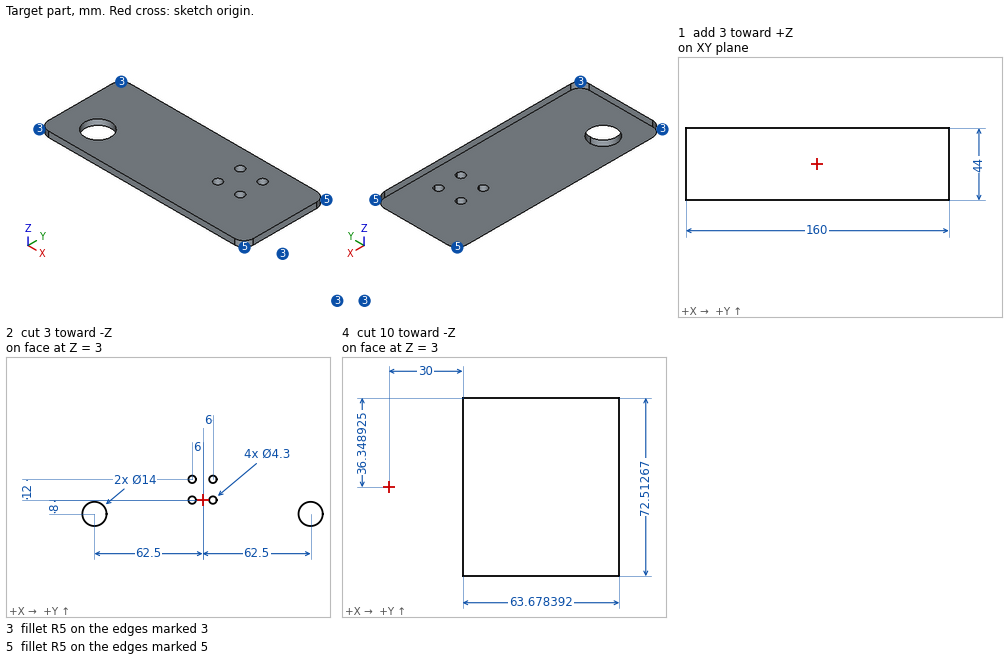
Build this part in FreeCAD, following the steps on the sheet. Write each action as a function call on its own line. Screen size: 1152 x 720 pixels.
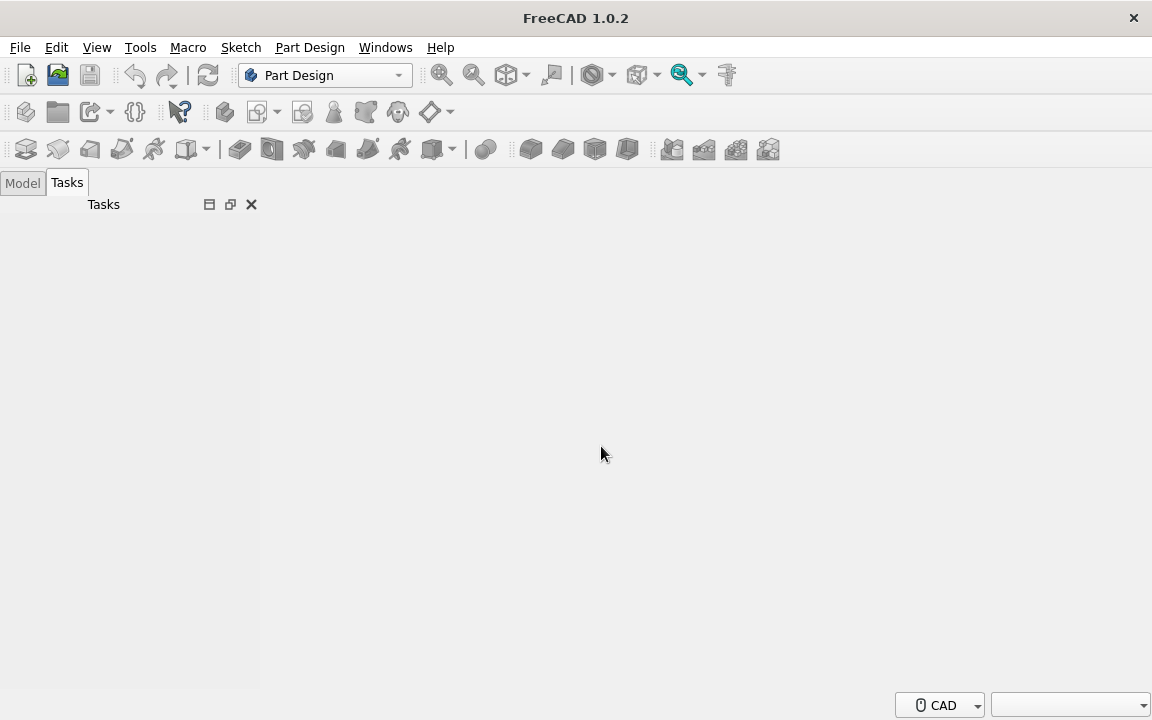
key(ctrl+n)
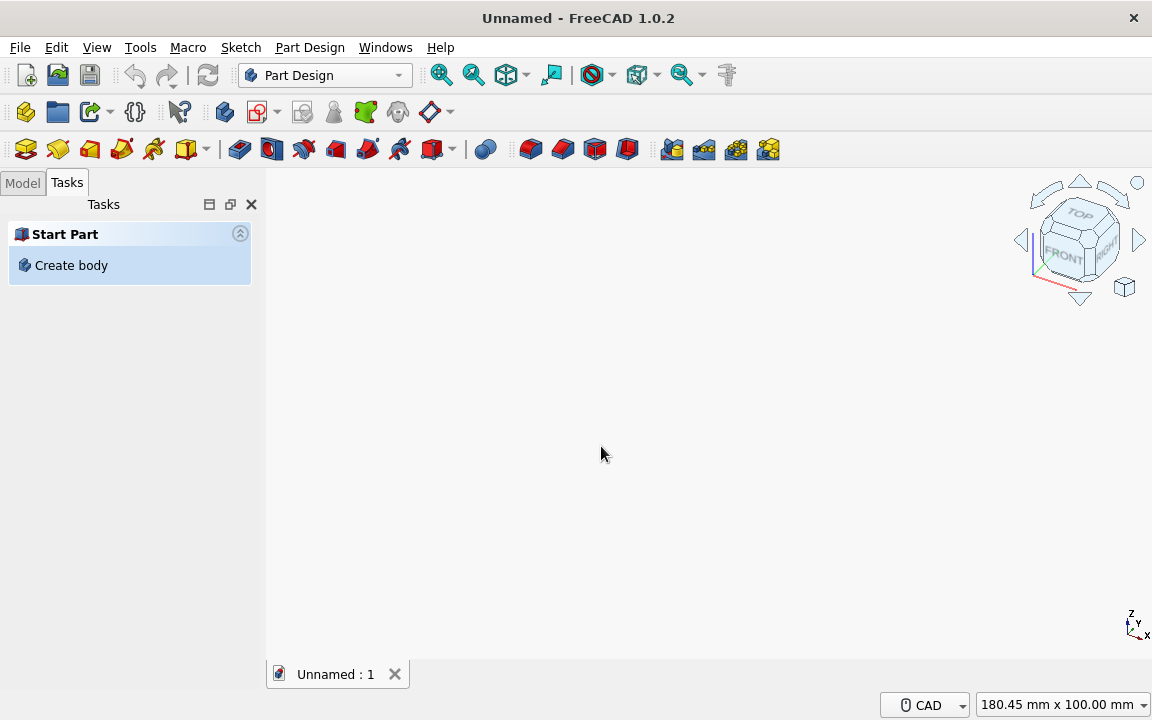
click(258, 112)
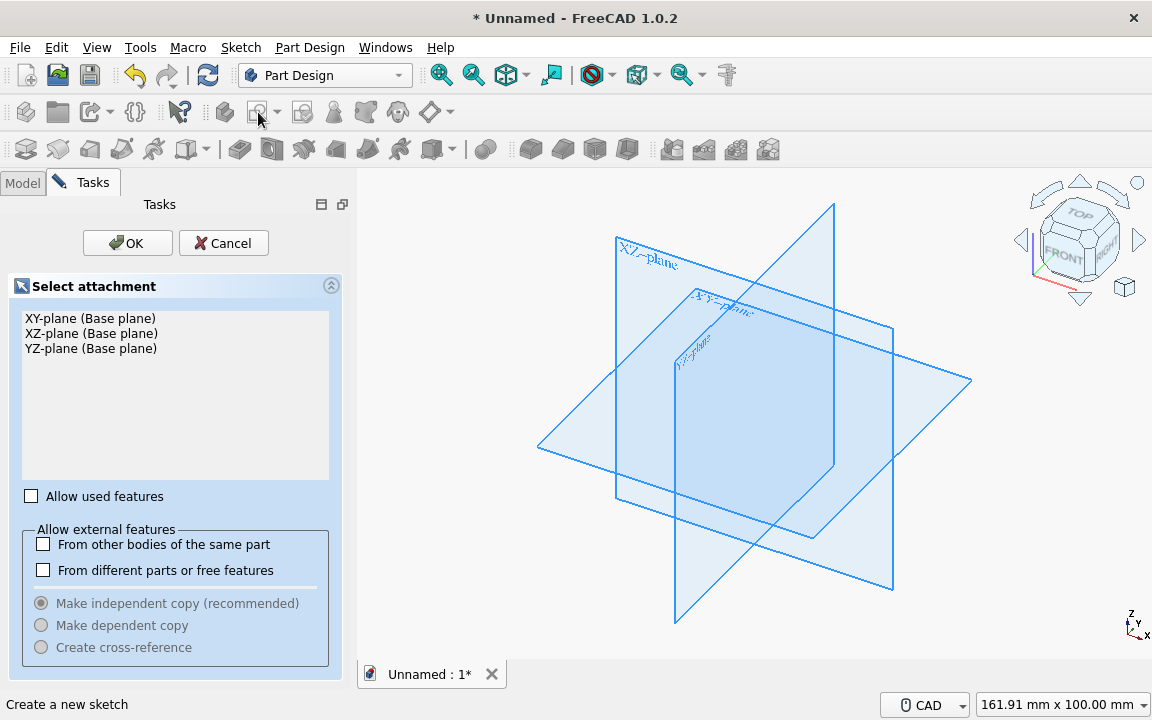
click(82, 318)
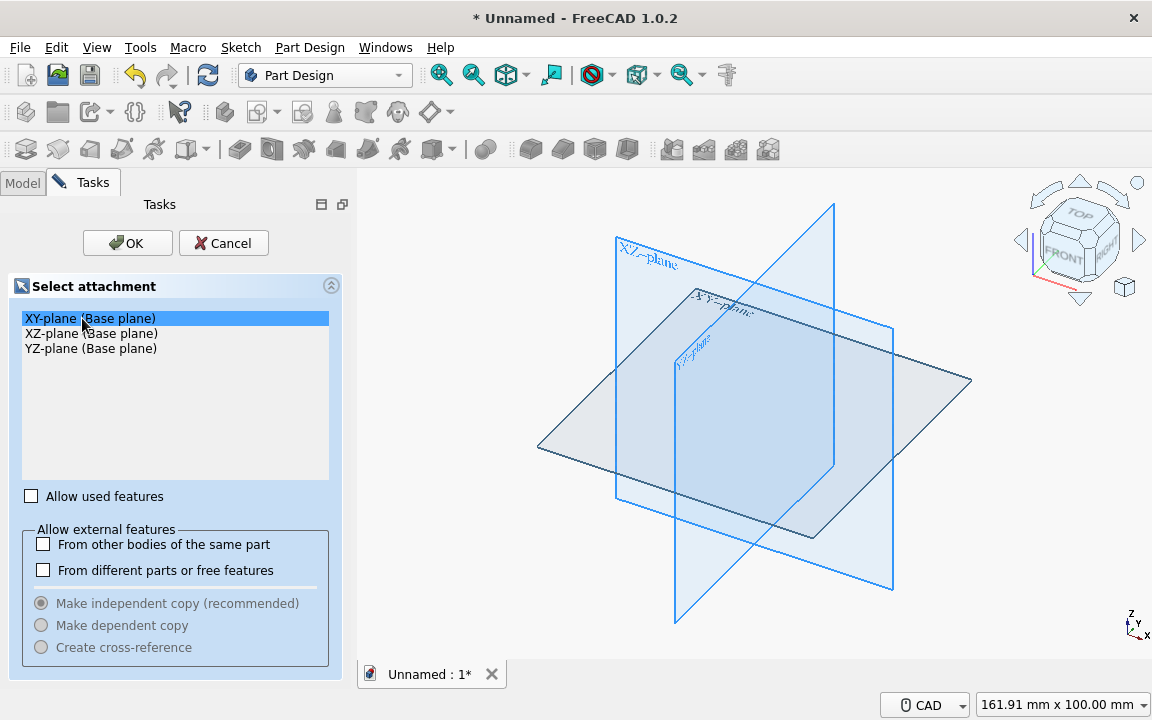
click(128, 243)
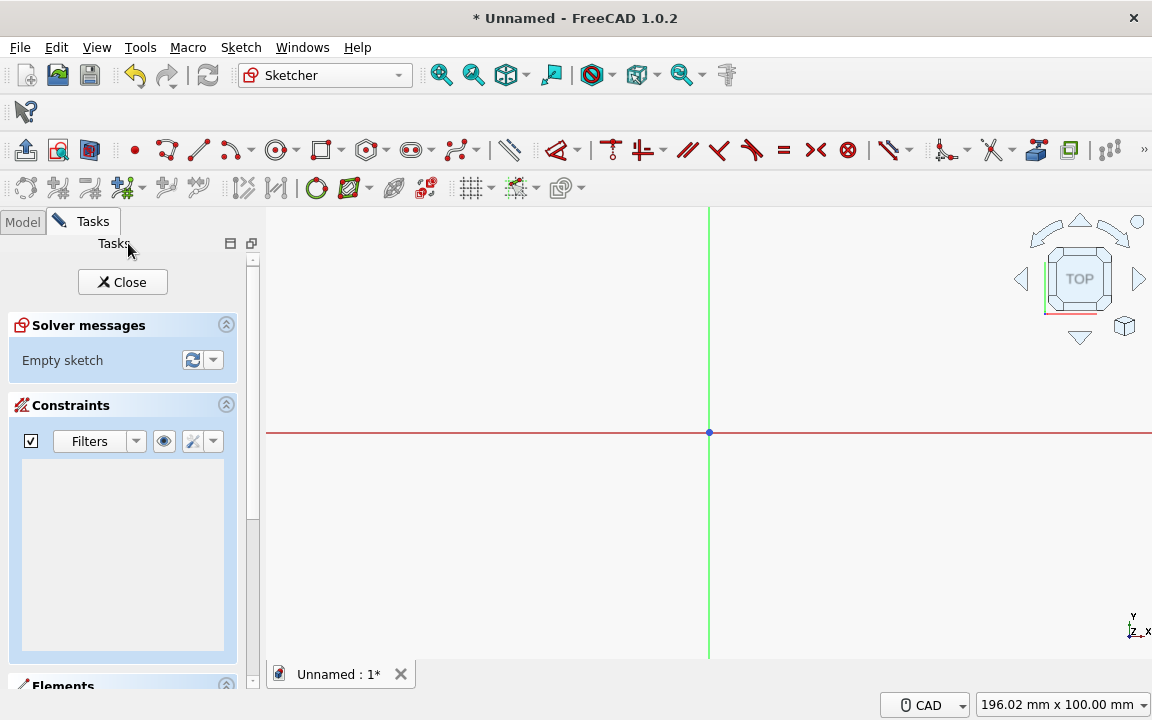
scroll(501, 433, down, 2)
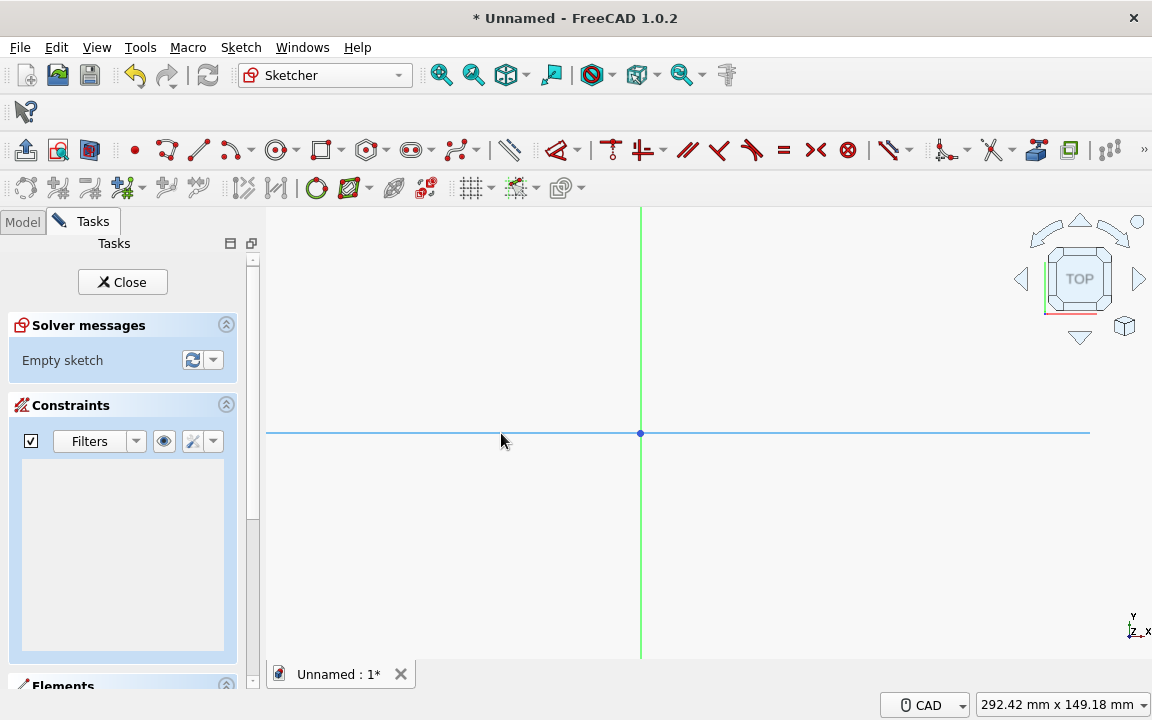
key(g)
key(v)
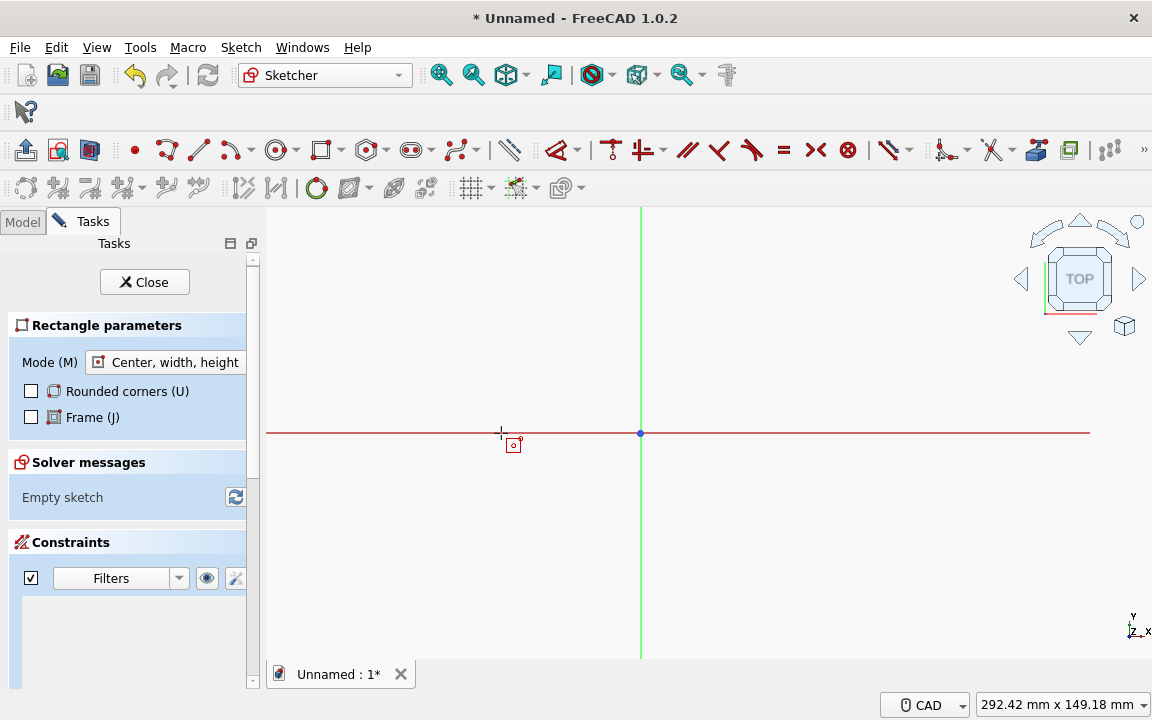
click(641, 433)
move(883, 367)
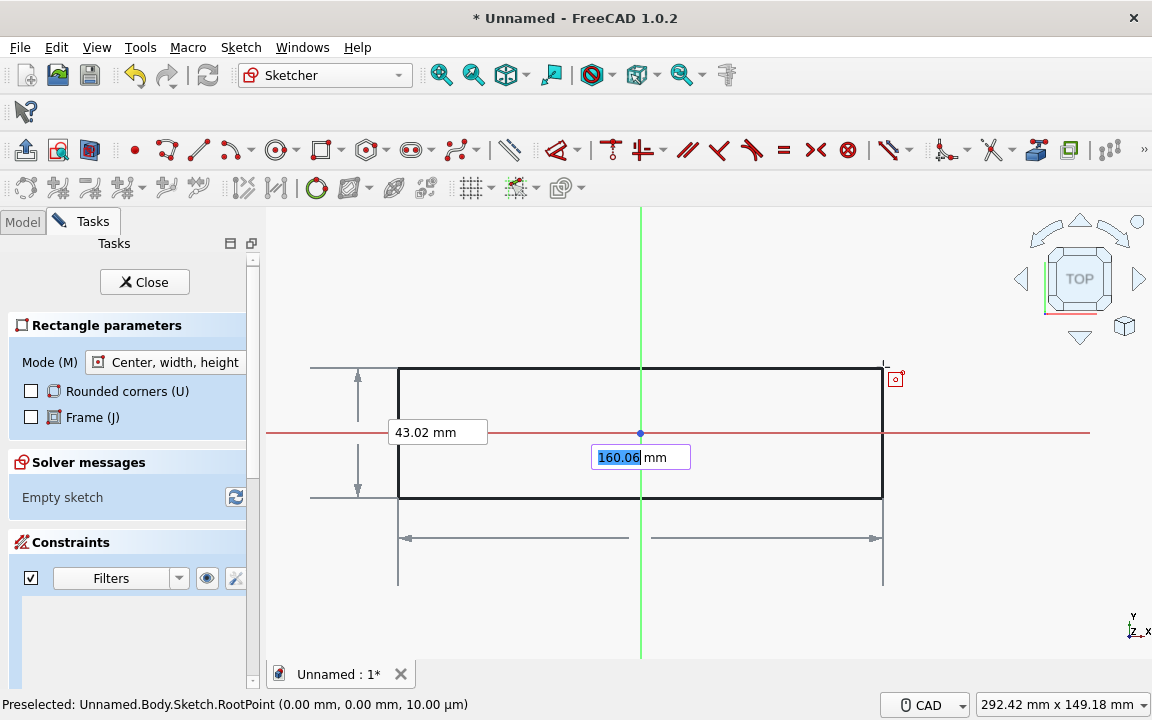
text(160)
key(Tab)
text(44)
key(Return)
key(Escape)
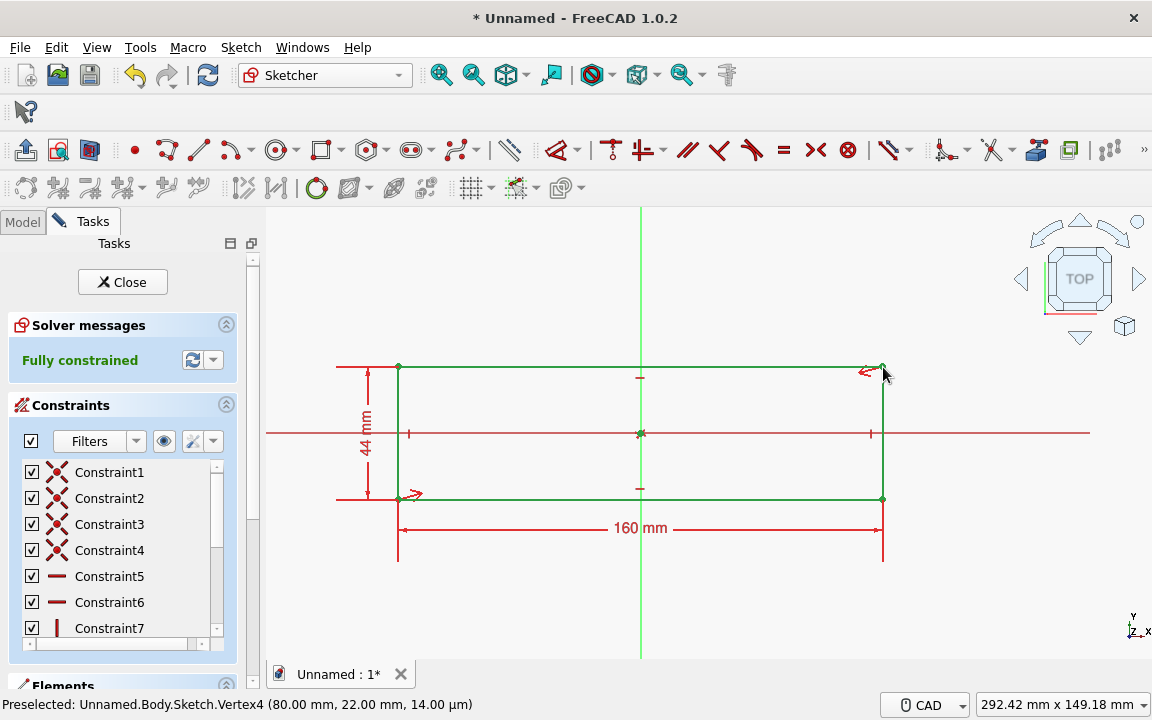
click(123, 282)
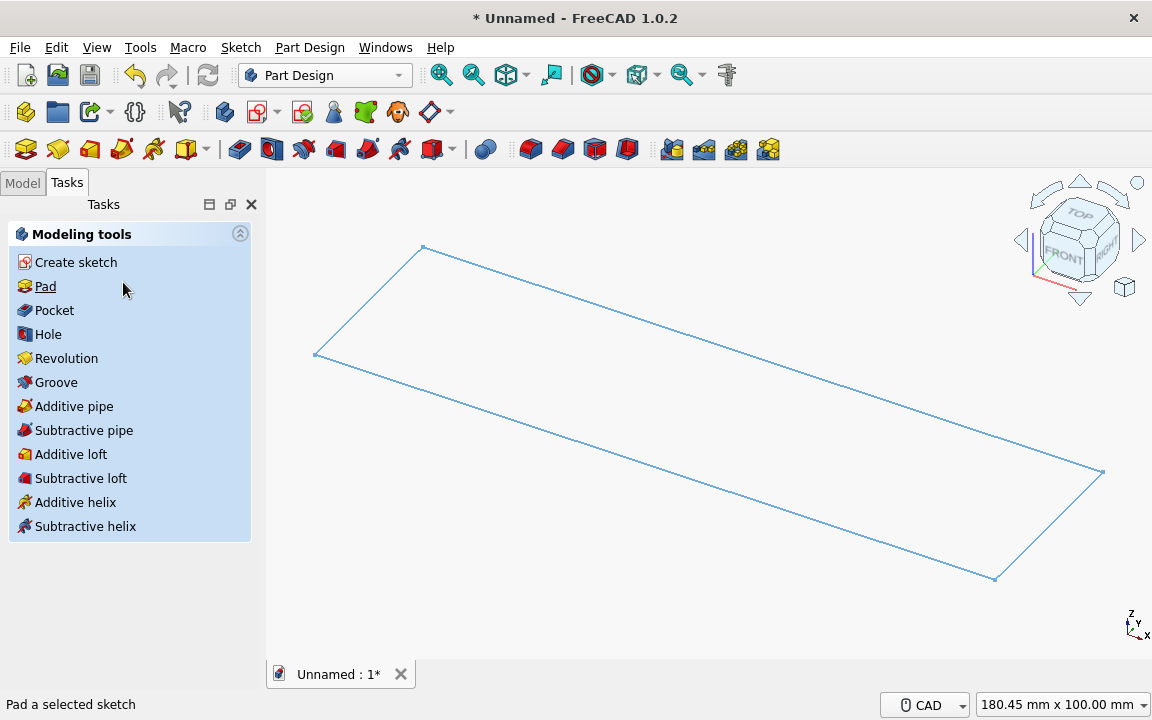
click(26, 150)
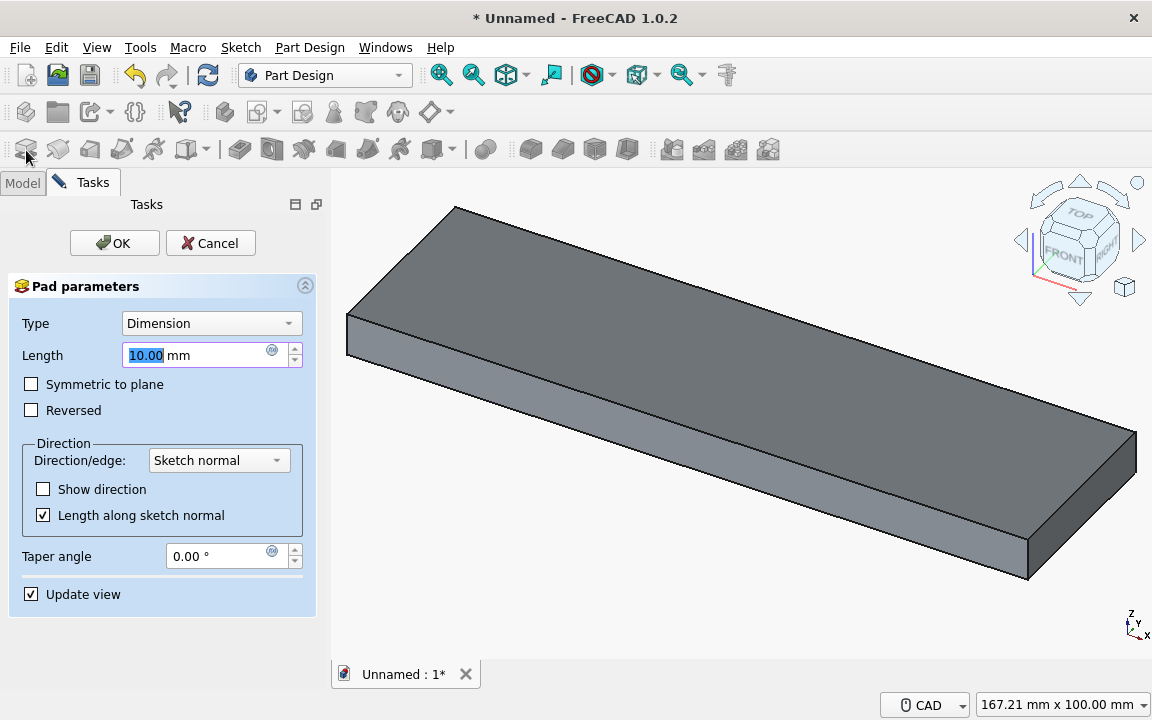
text(3)
key(Tab)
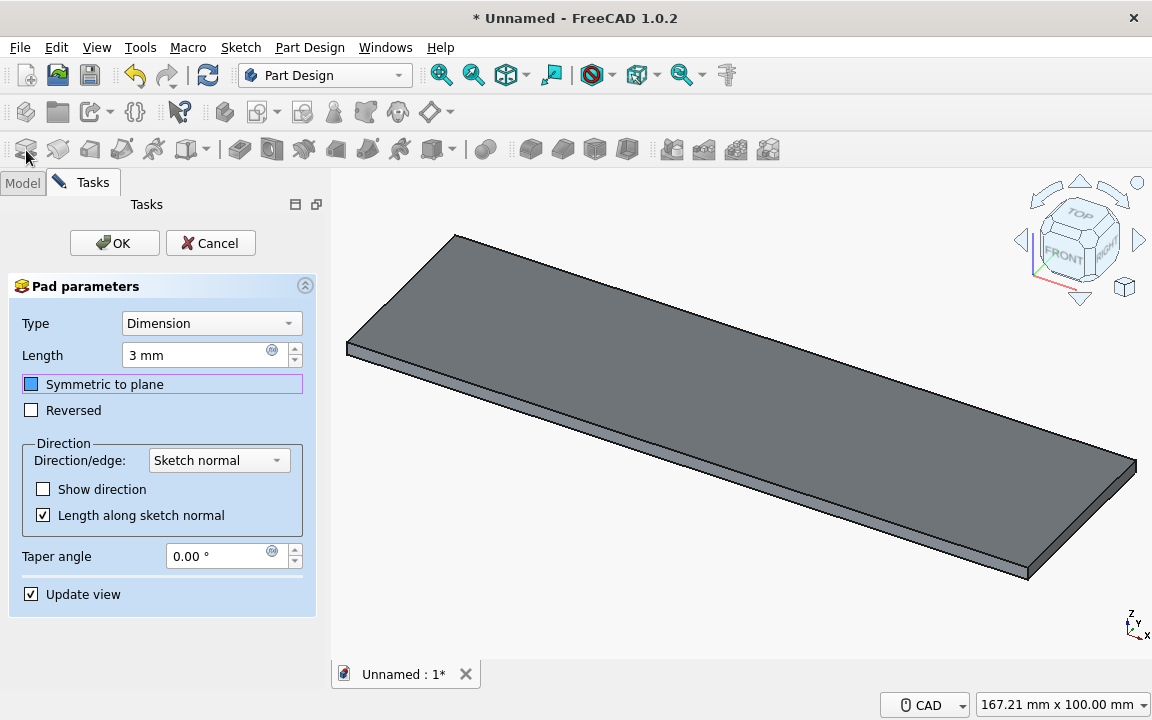
click(115, 243)